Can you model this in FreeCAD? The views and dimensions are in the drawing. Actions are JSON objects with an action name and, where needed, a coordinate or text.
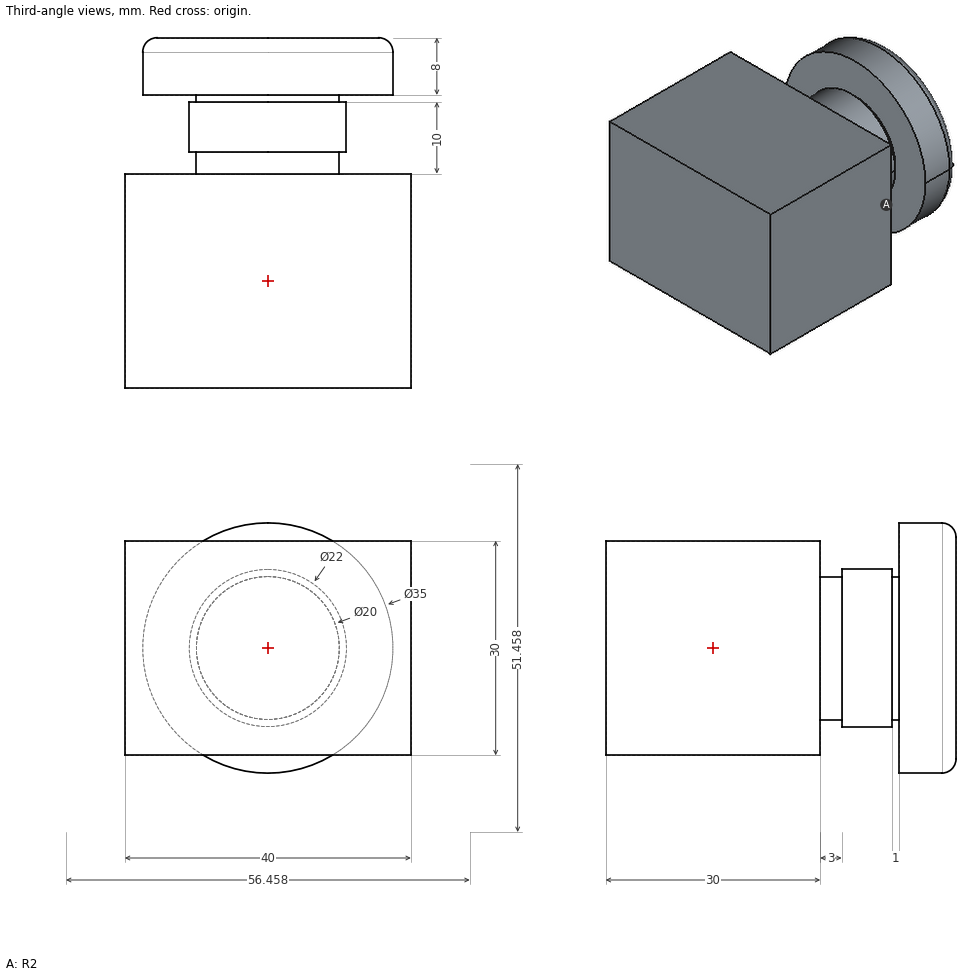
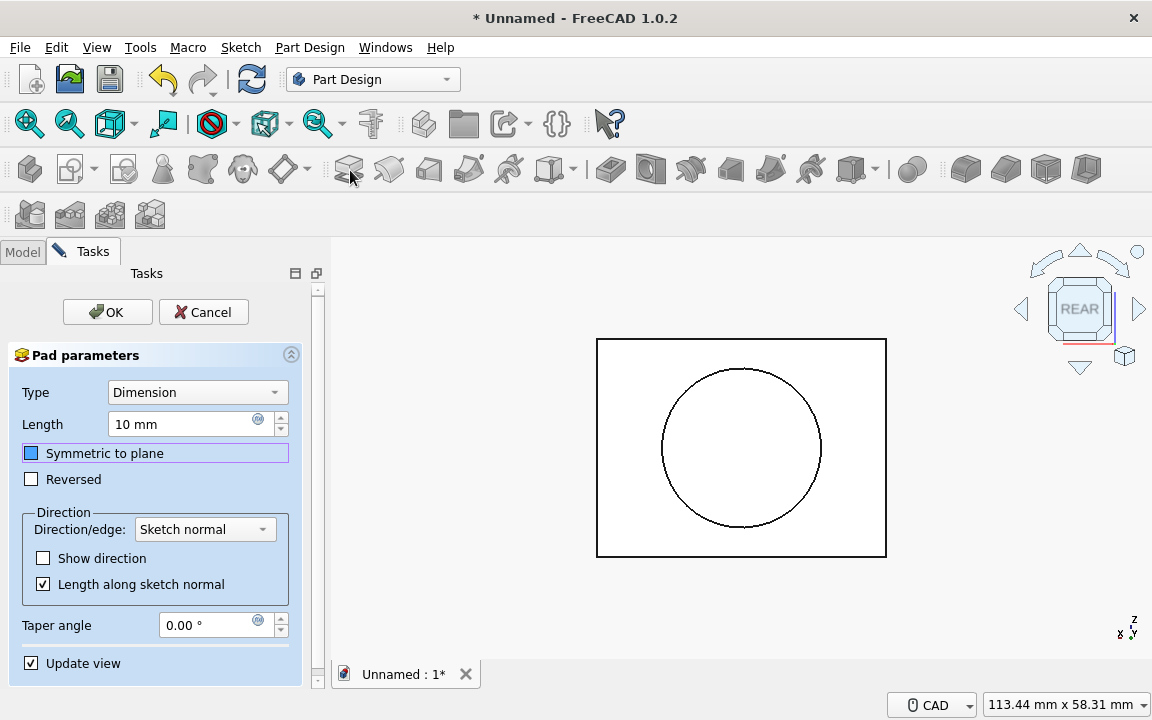
{"action": "left_click", "coordinate": [108, 312]}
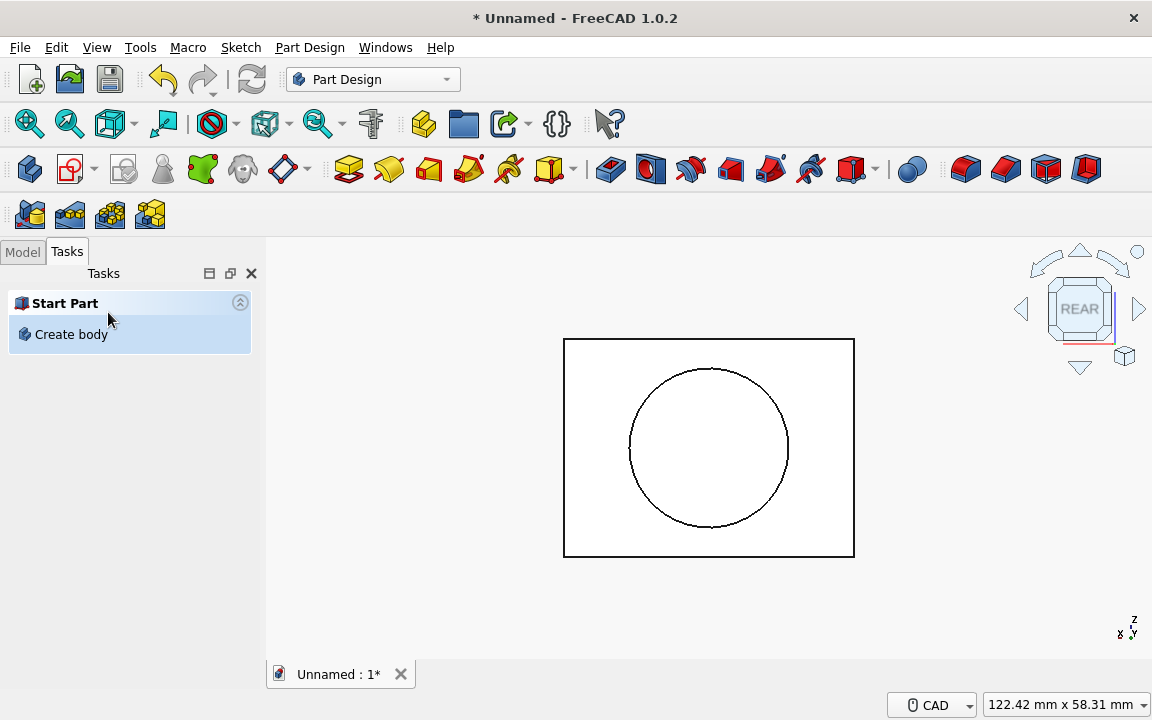
{"action": "left_click", "coordinate": [709, 447]}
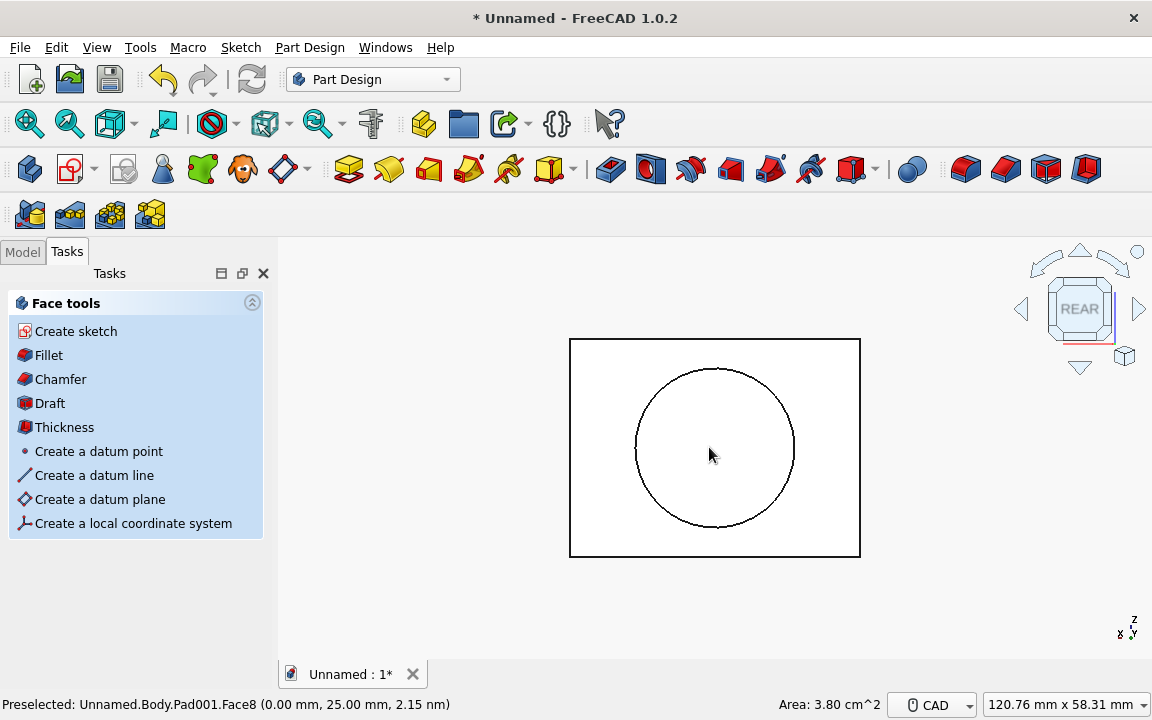
{"action": "left_click", "coordinate": [70, 170]}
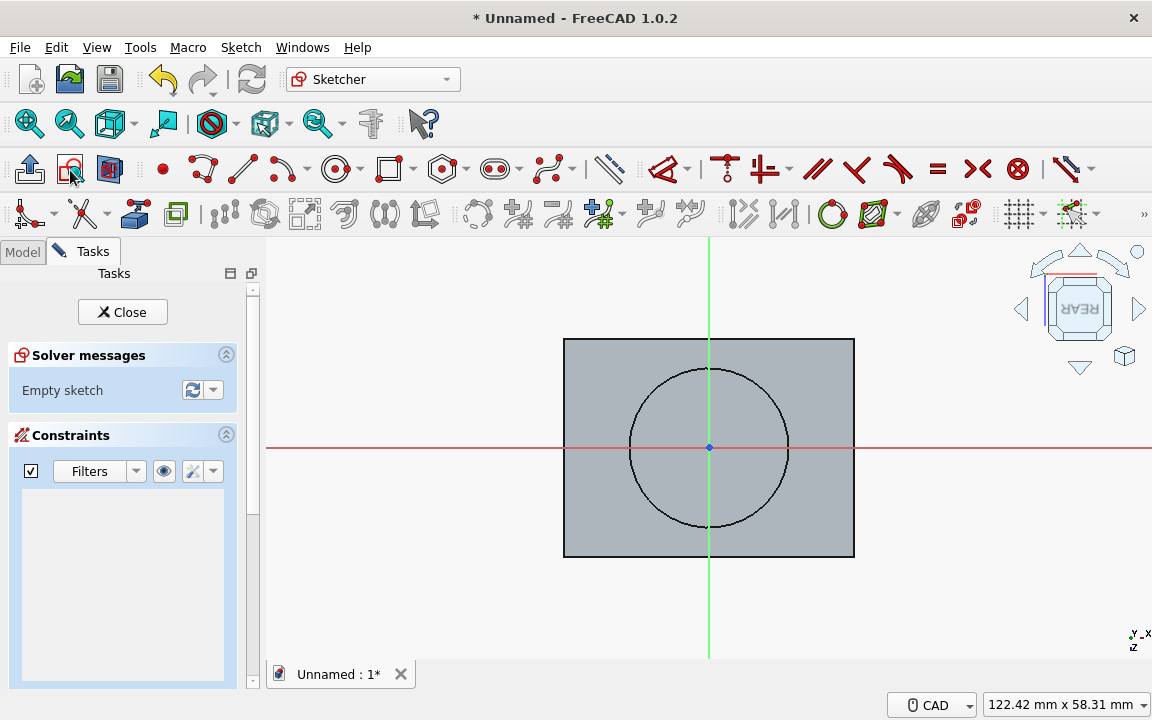
{"action": "scroll", "coordinate": [792, 448], "scroll_direction": "up", "scroll_amount": 3}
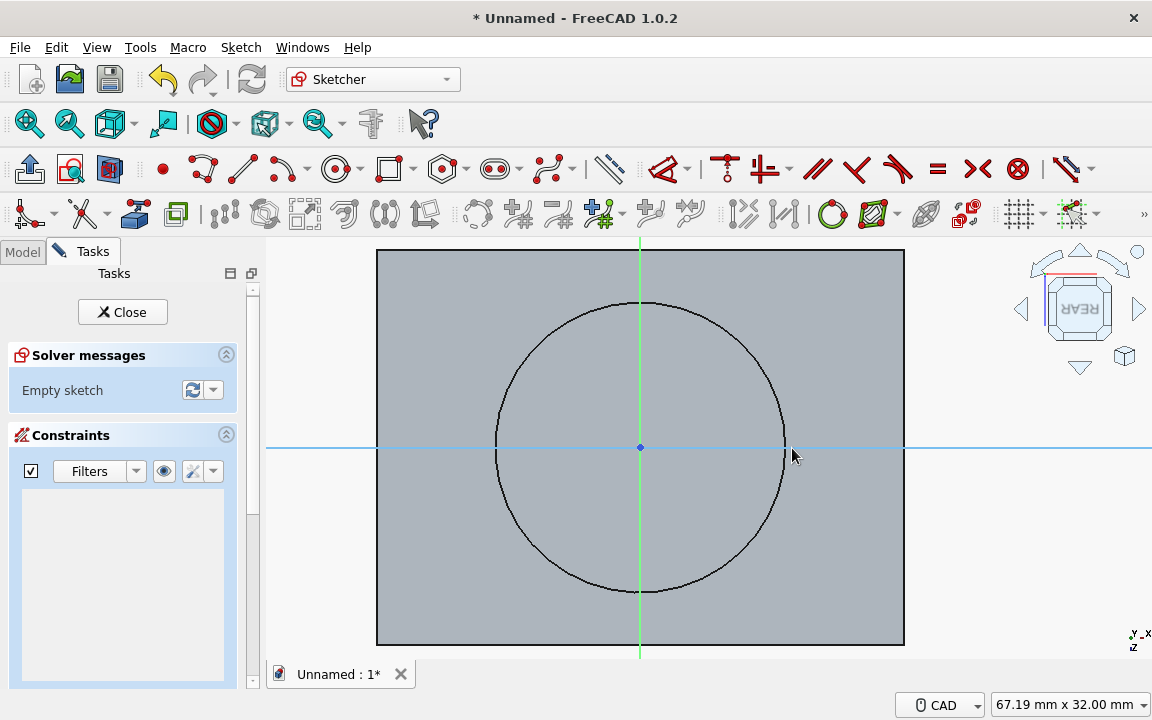
{"action": "left_click", "coordinate": [336, 170]}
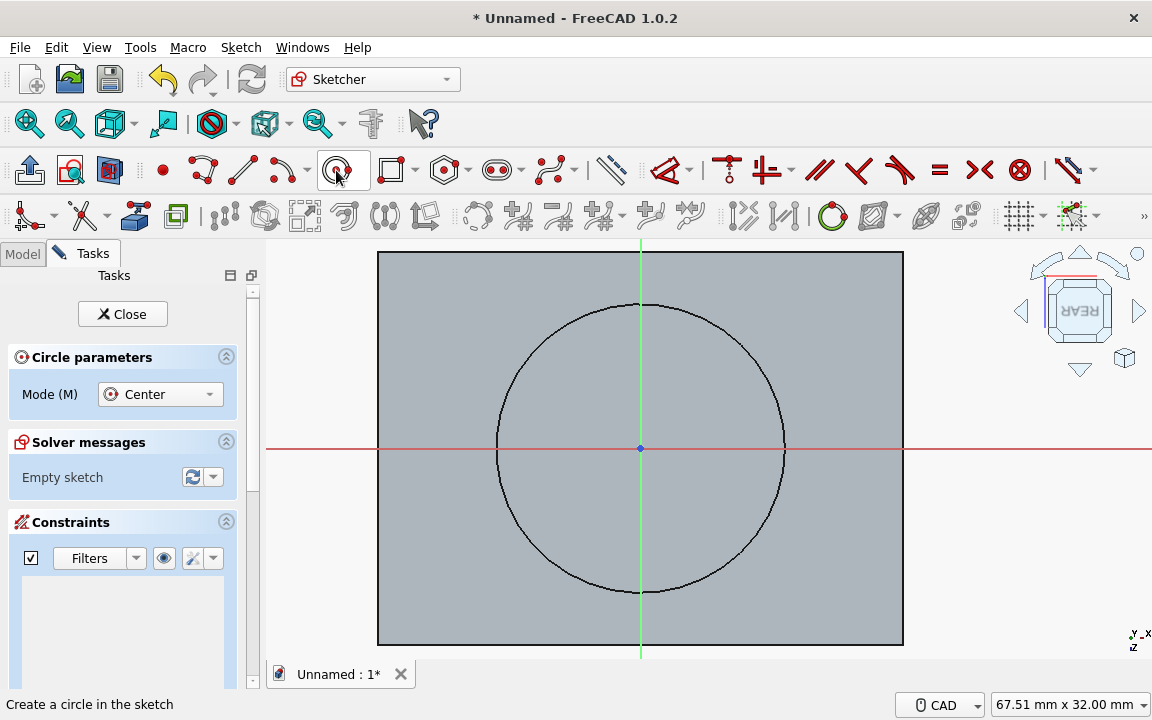
{"action": "left_click", "coordinate": [641, 449]}
{"action": "mouse_move", "coordinate": [733, 356]}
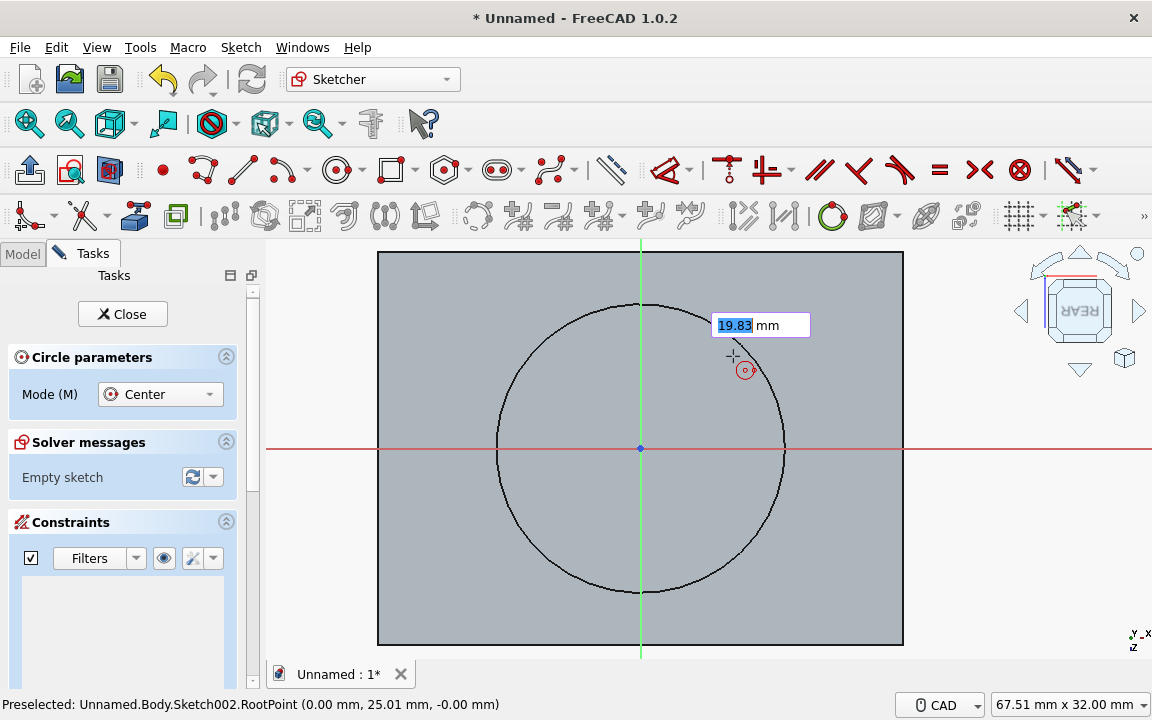
{"action": "type", "text": "20"}
{"action": "key", "text": "Return"}
{"action": "key", "text": "Escape"}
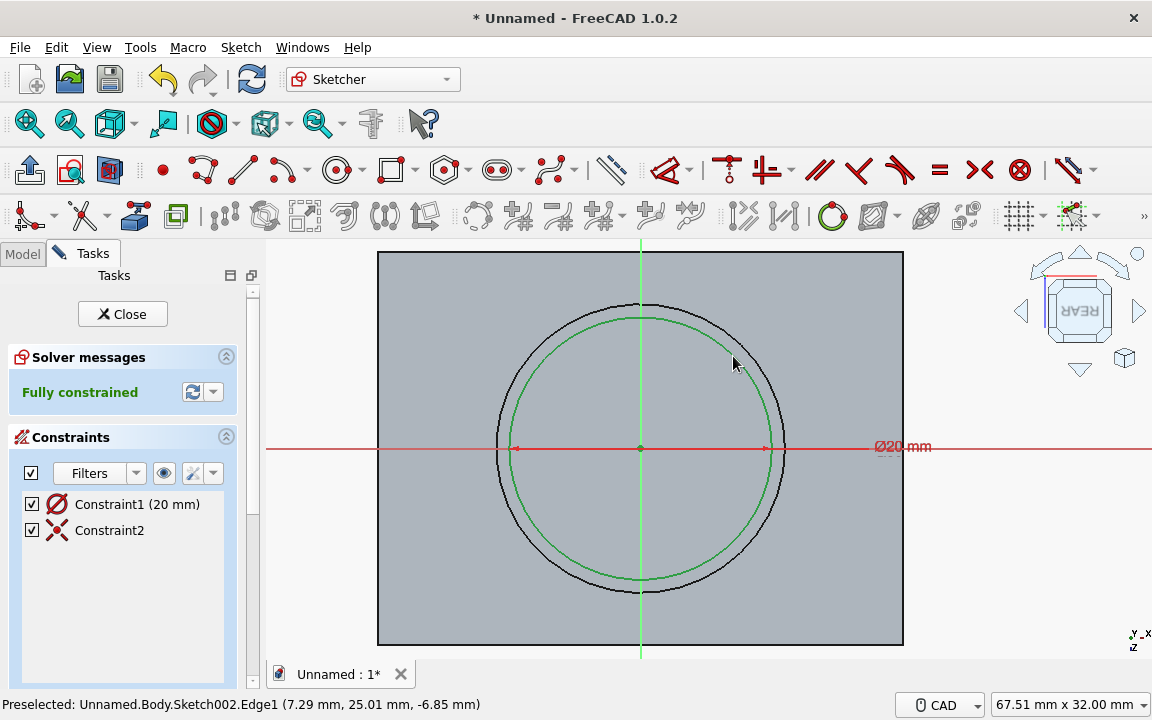
{"action": "left_click", "coordinate": [123, 314]}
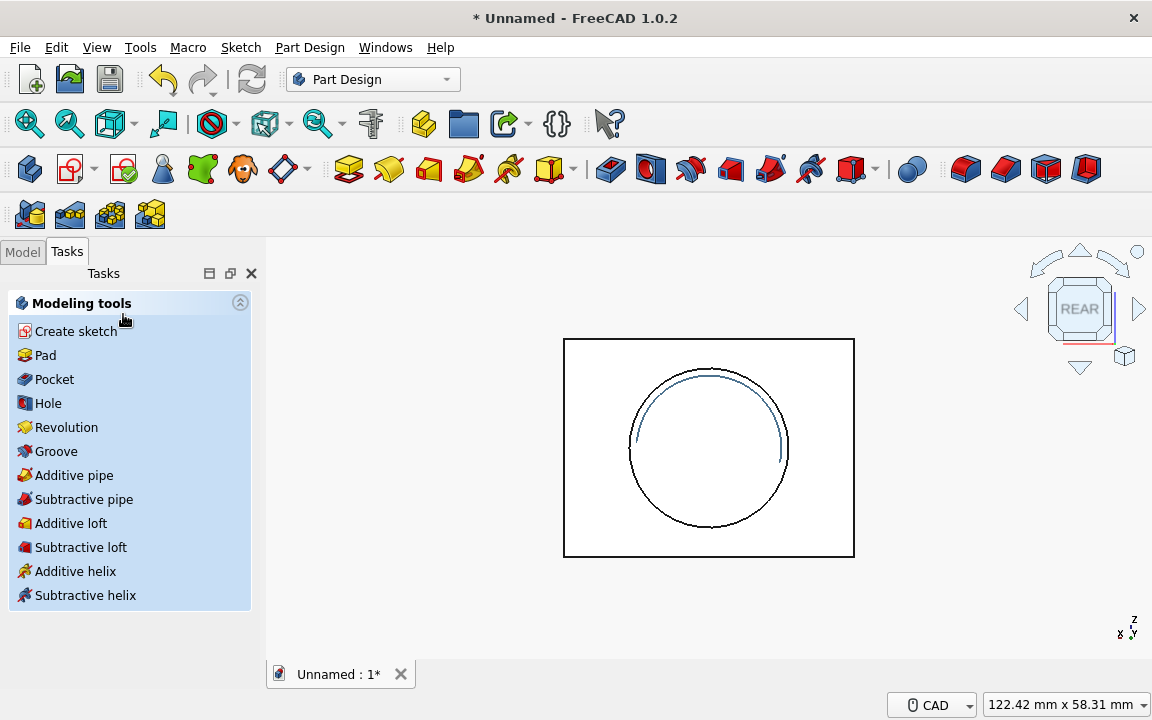
{"action": "left_click", "coordinate": [350, 170]}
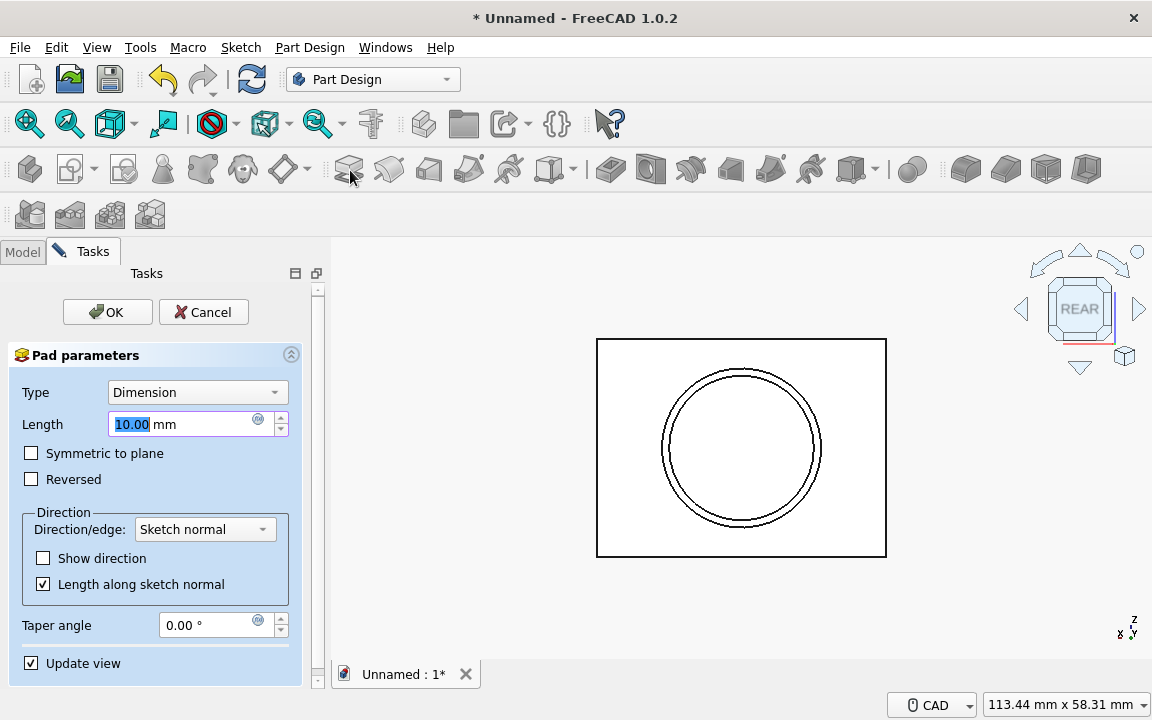
{"action": "type", "text": "1"}
{"action": "key", "text": "Tab"}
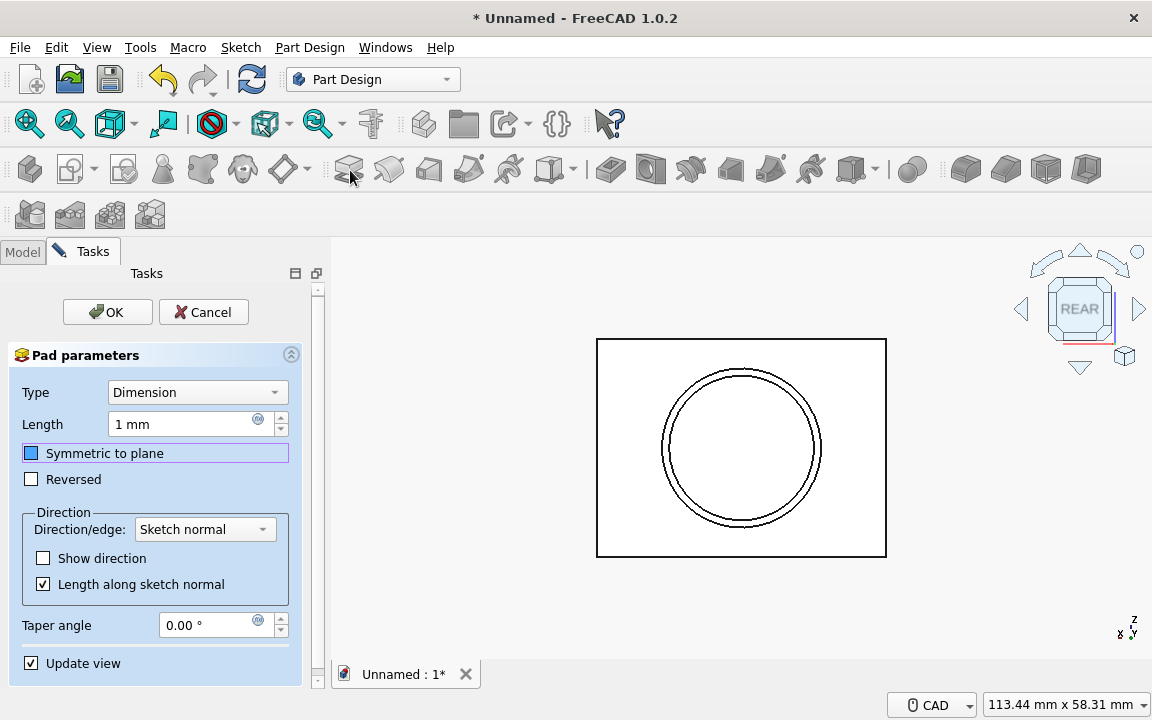
{"action": "left_click", "coordinate": [108, 312]}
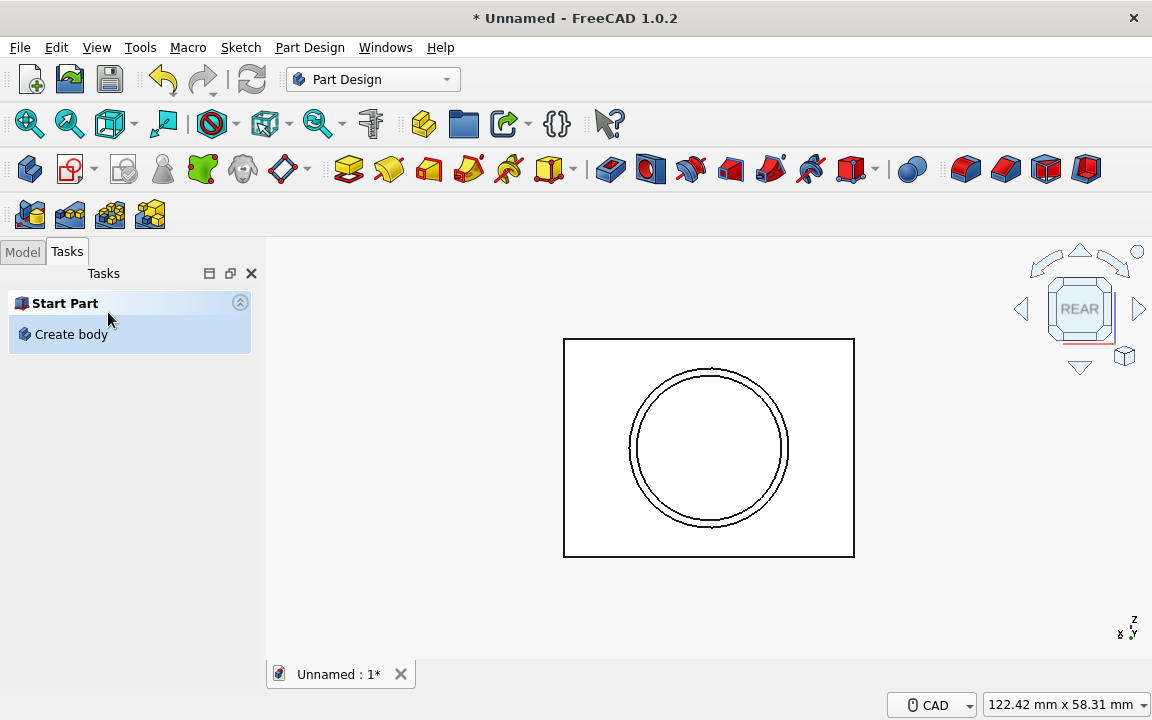
{"action": "left_click", "coordinate": [709, 447]}